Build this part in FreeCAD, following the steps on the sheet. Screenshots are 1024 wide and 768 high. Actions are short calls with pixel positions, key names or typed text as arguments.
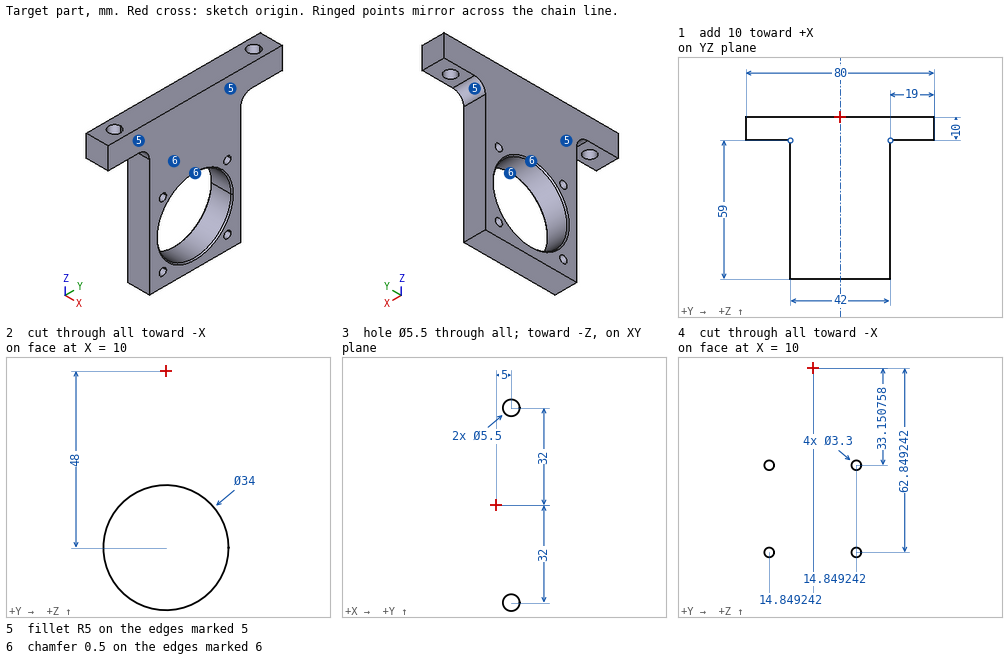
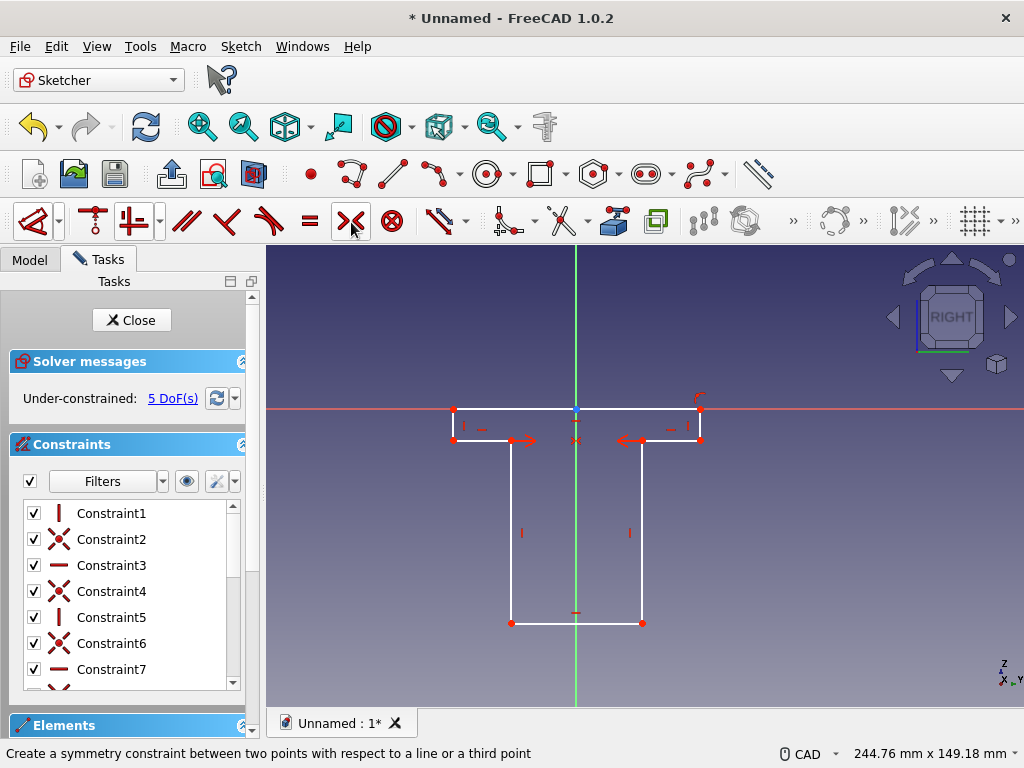
click(511, 496)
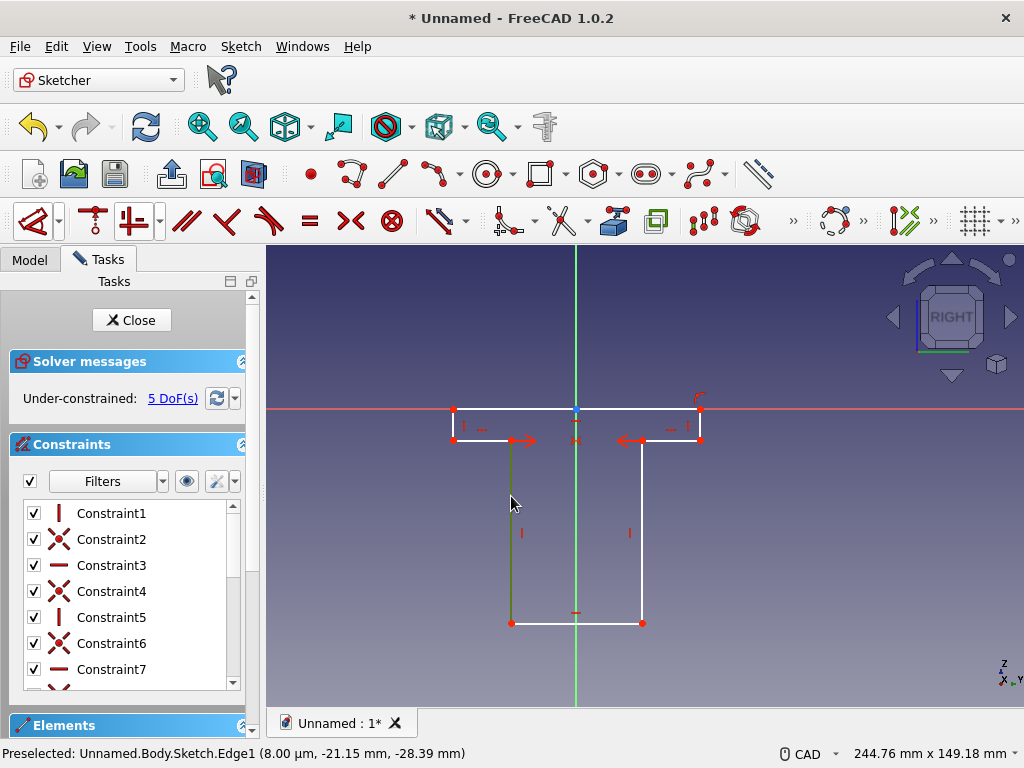
key(i)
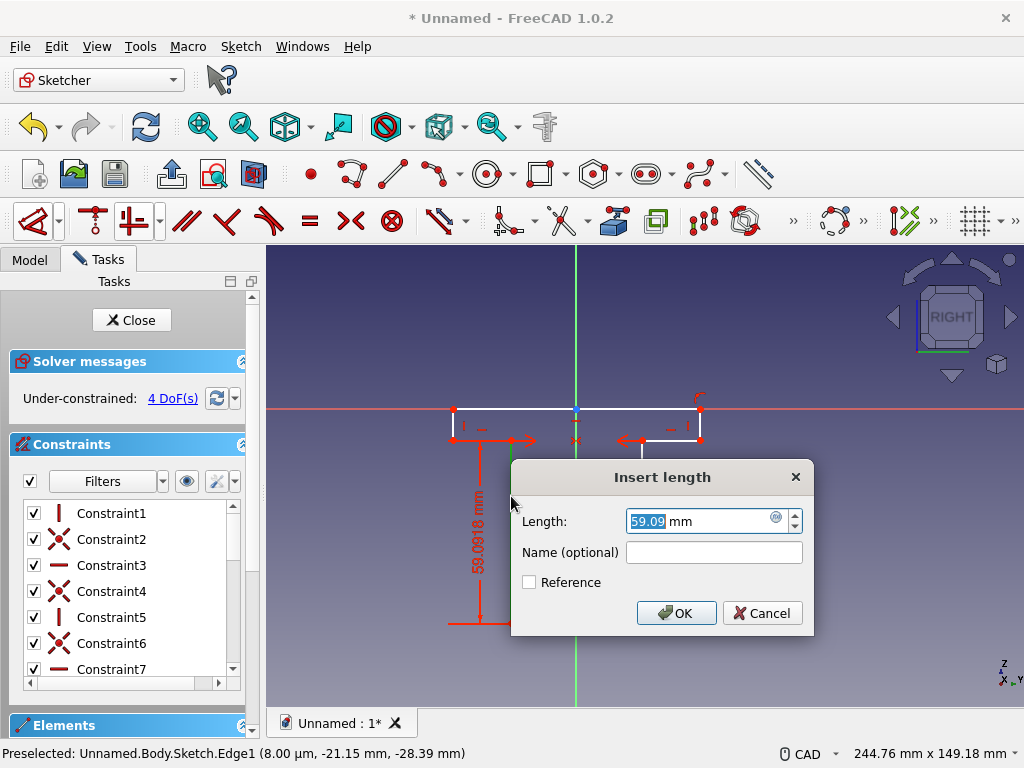
text(59)
key(Return)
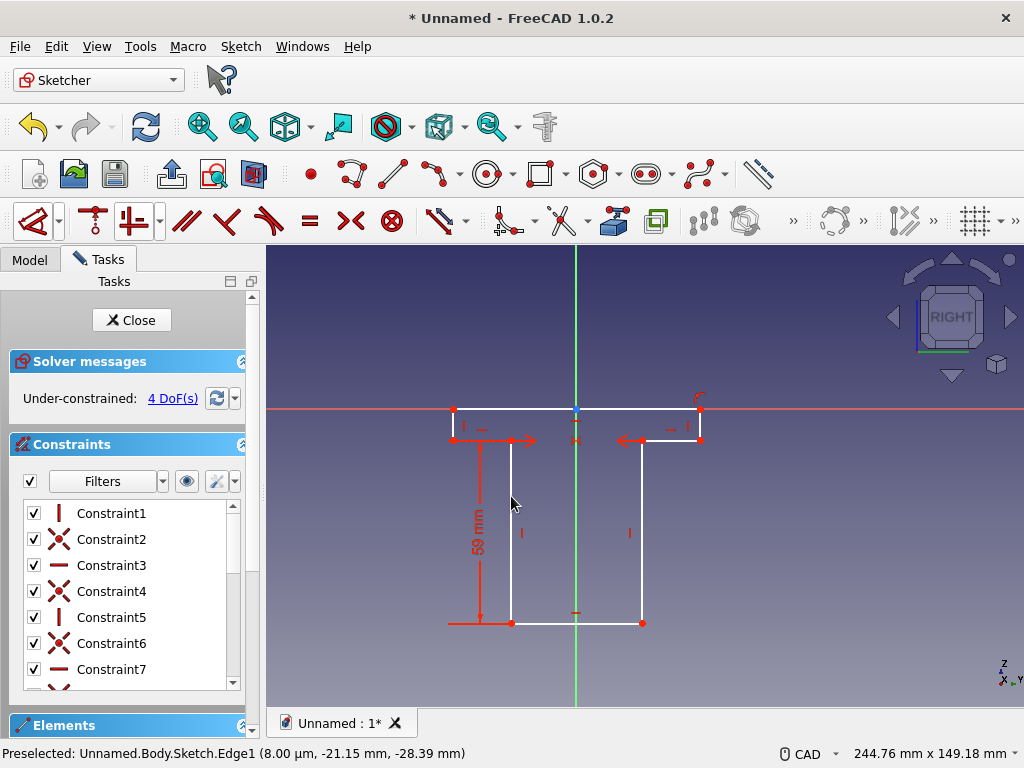
click(550, 624)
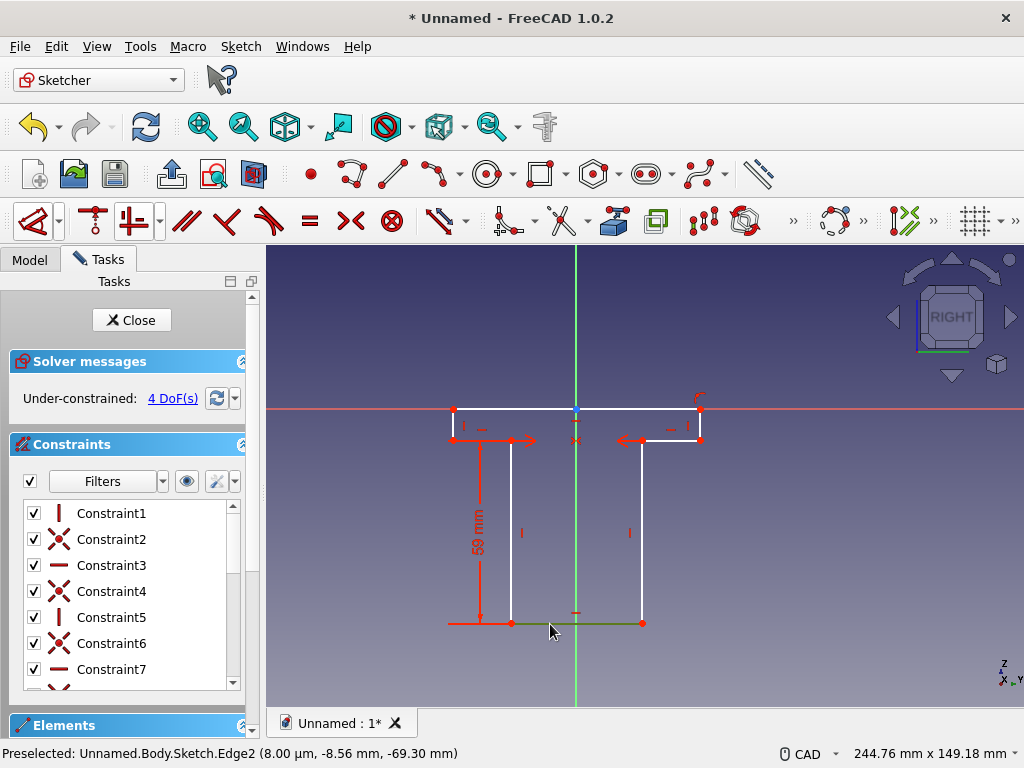
click(58, 222)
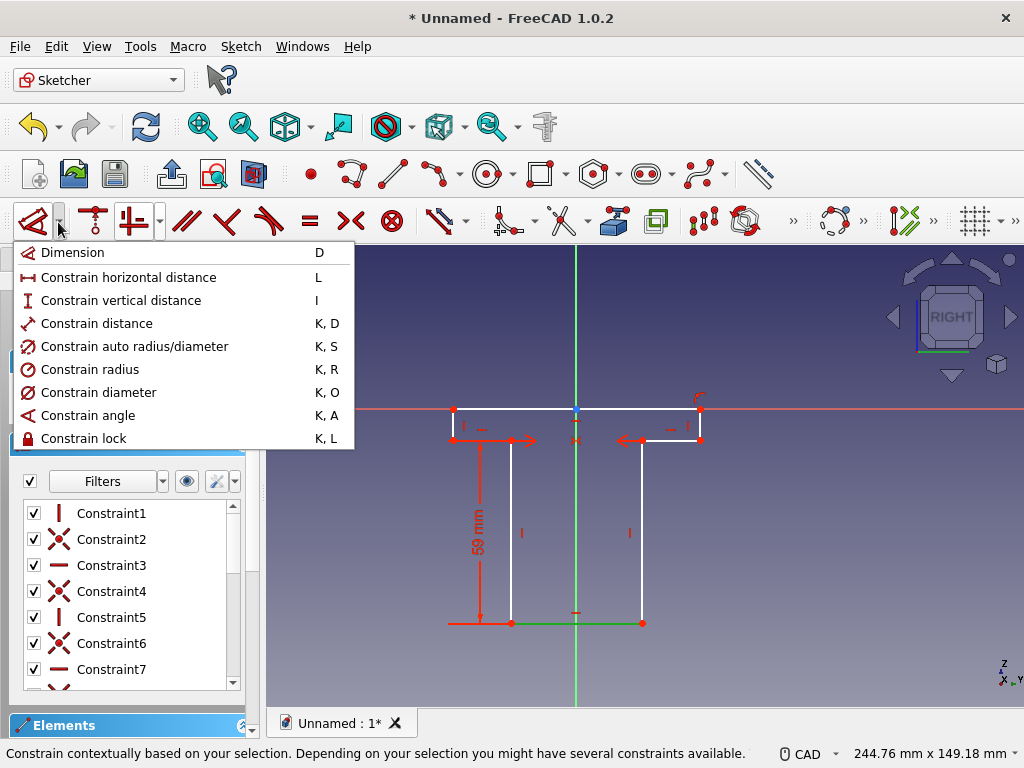
click(184, 278)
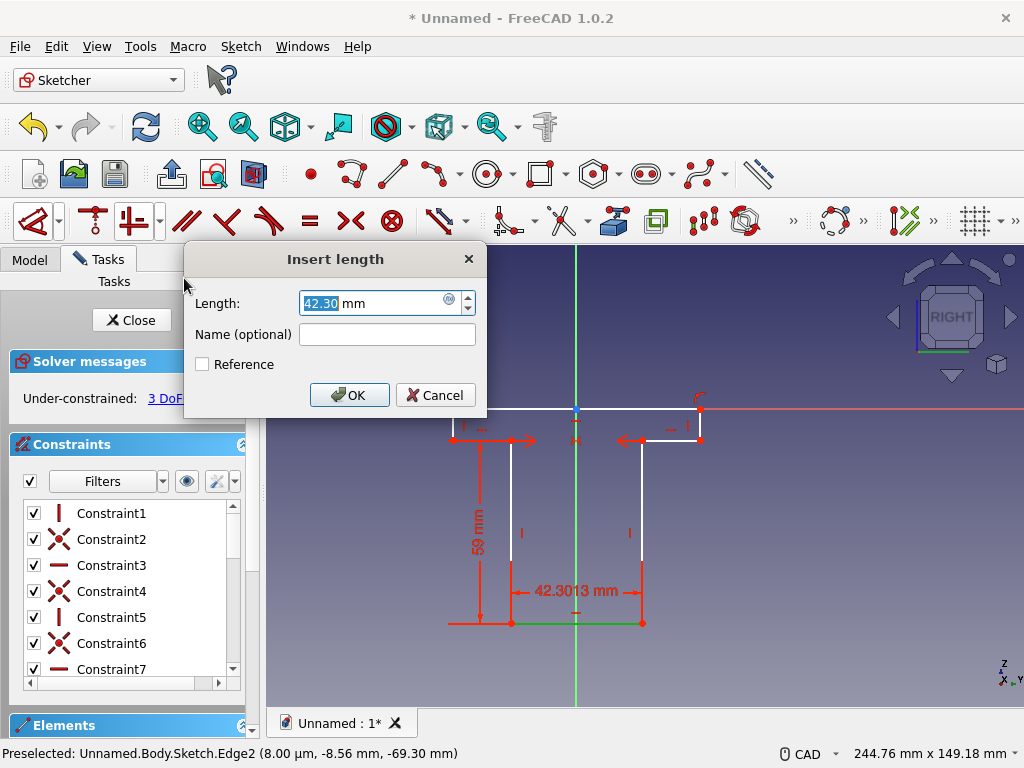
text(42)
key(Return)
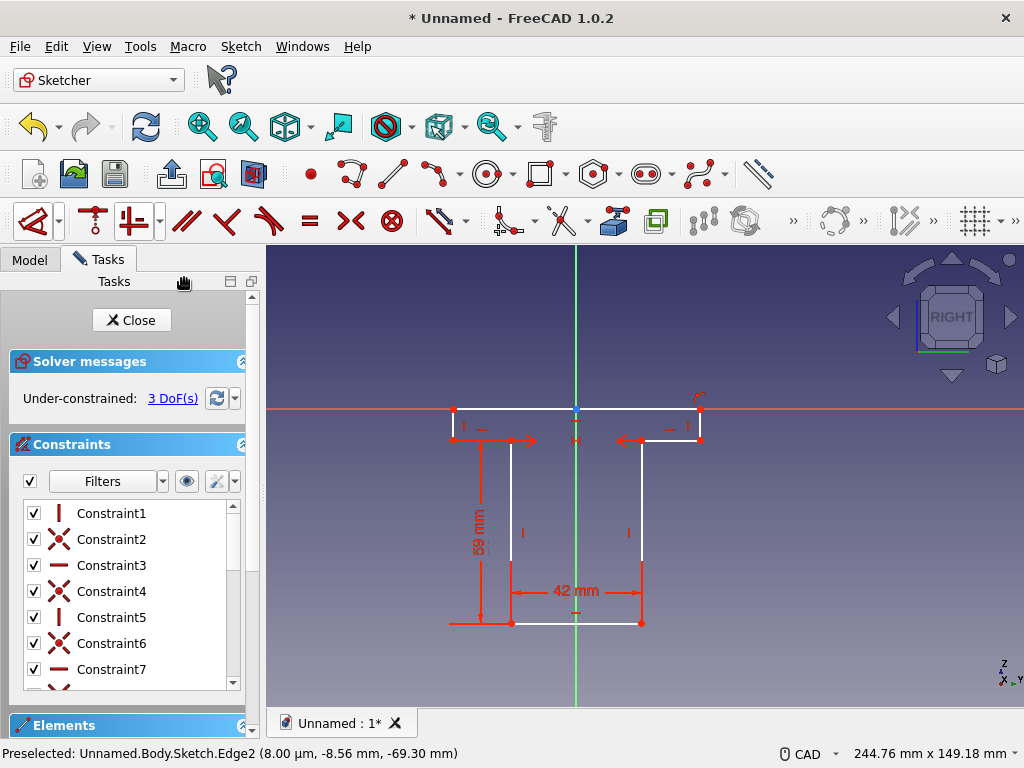
click(659, 441)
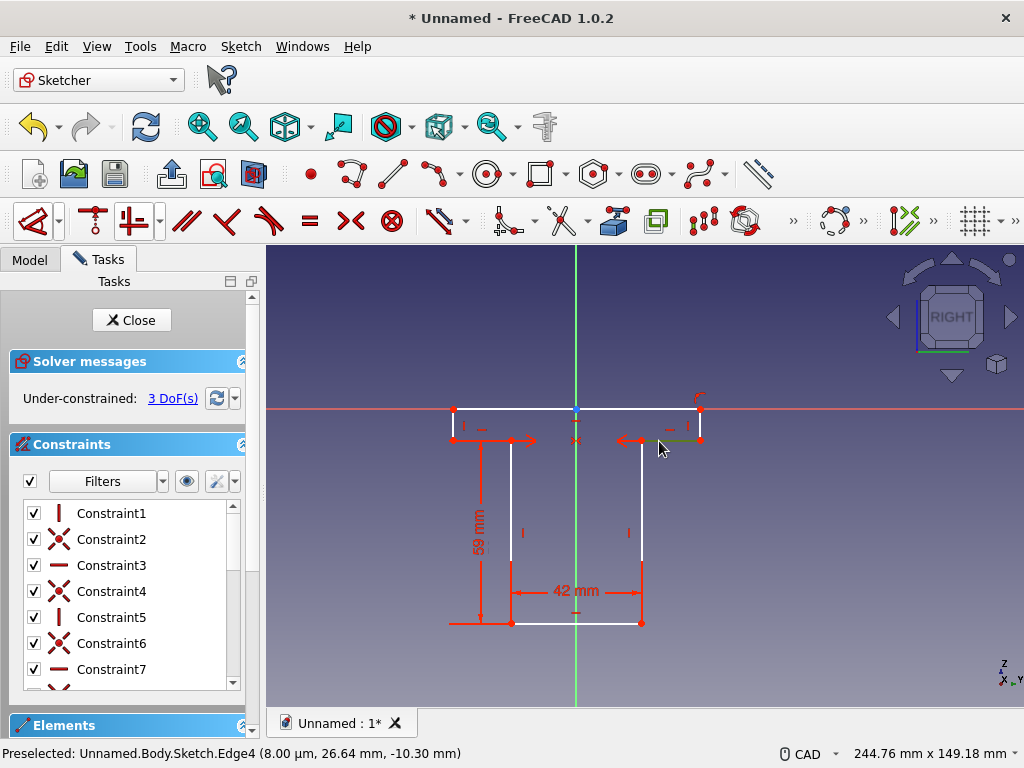
click(58, 222)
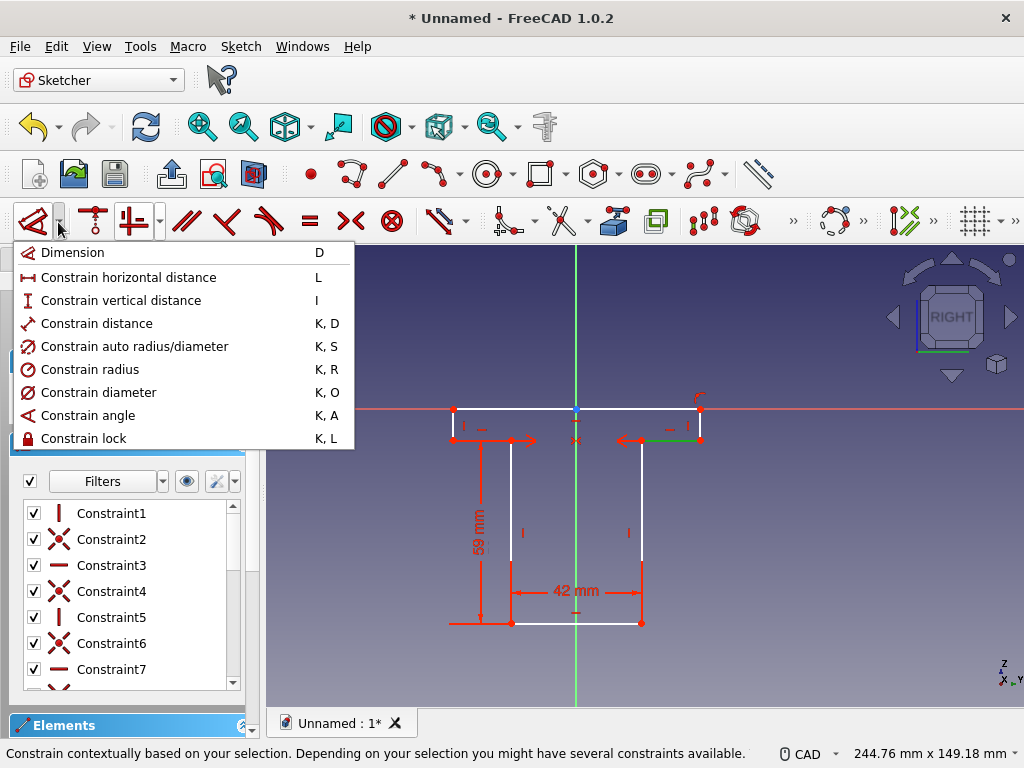
click(184, 278)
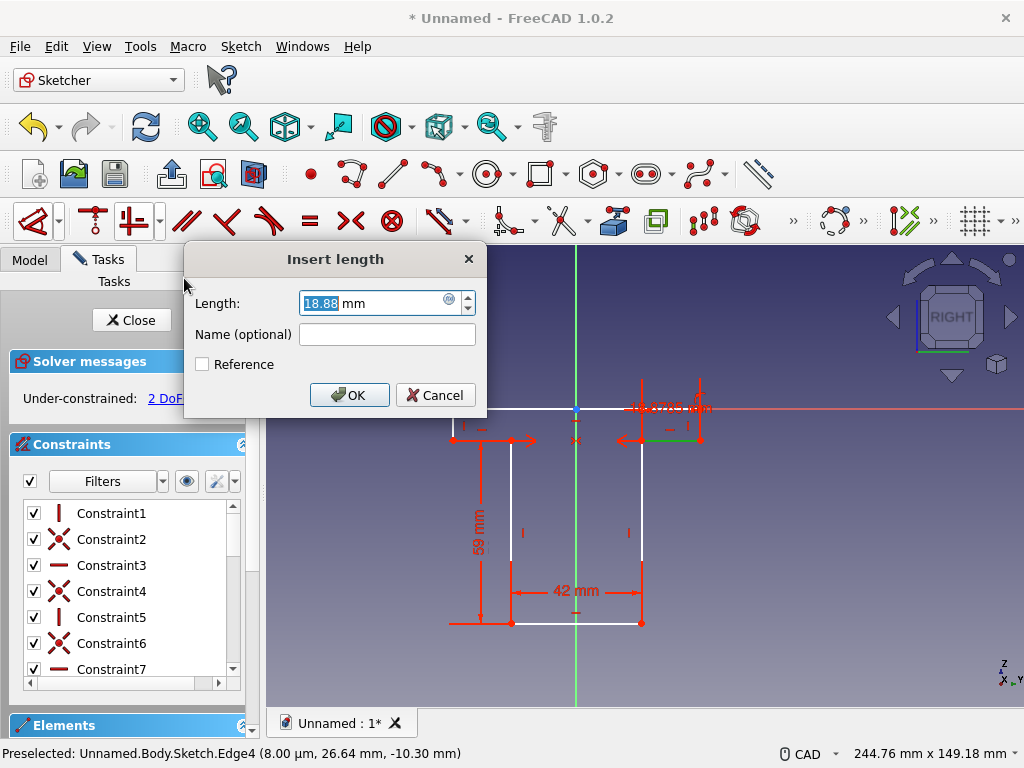
text(19)
key(Return)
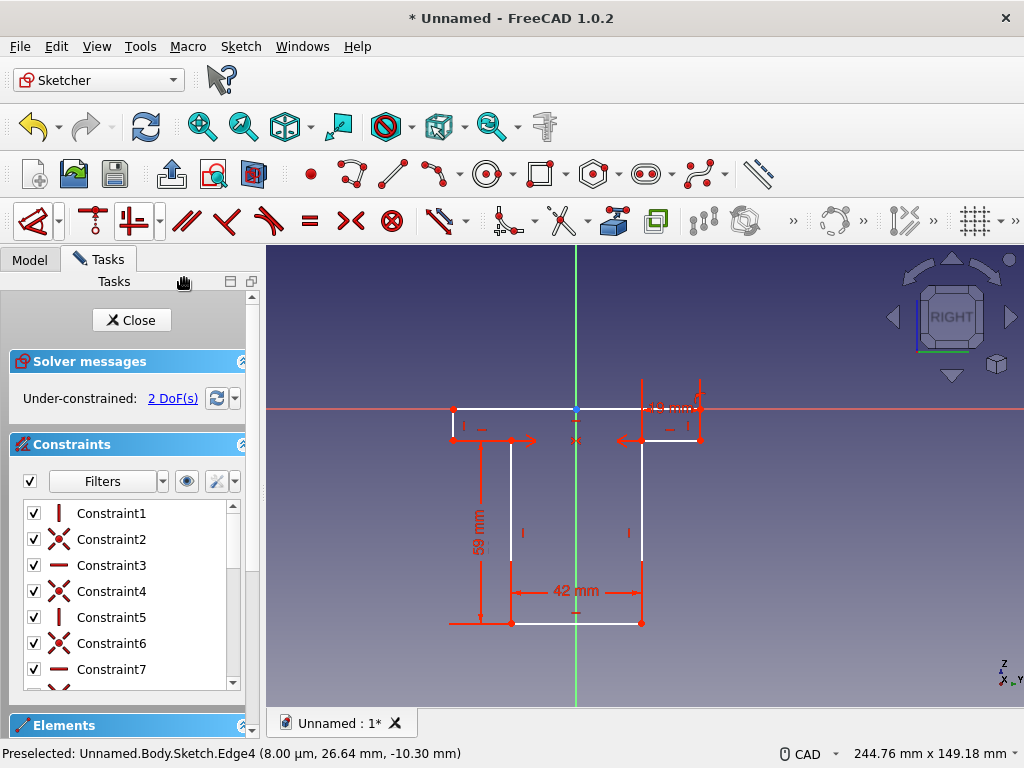
scroll(700, 431, up, 2)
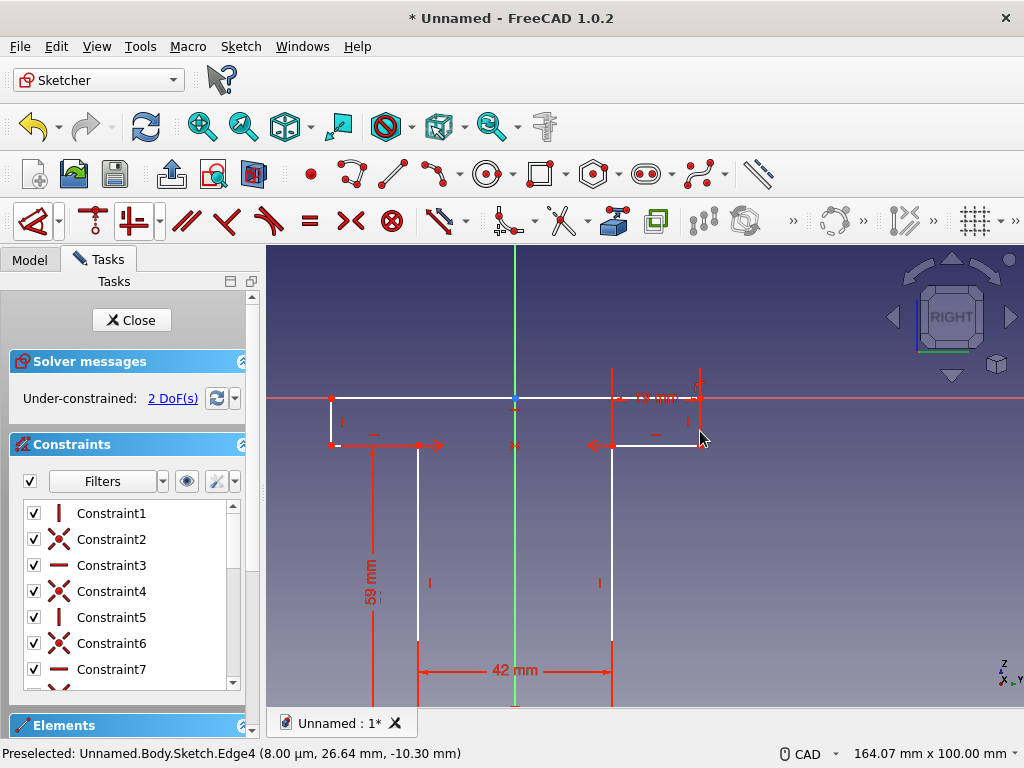
click(700, 431)